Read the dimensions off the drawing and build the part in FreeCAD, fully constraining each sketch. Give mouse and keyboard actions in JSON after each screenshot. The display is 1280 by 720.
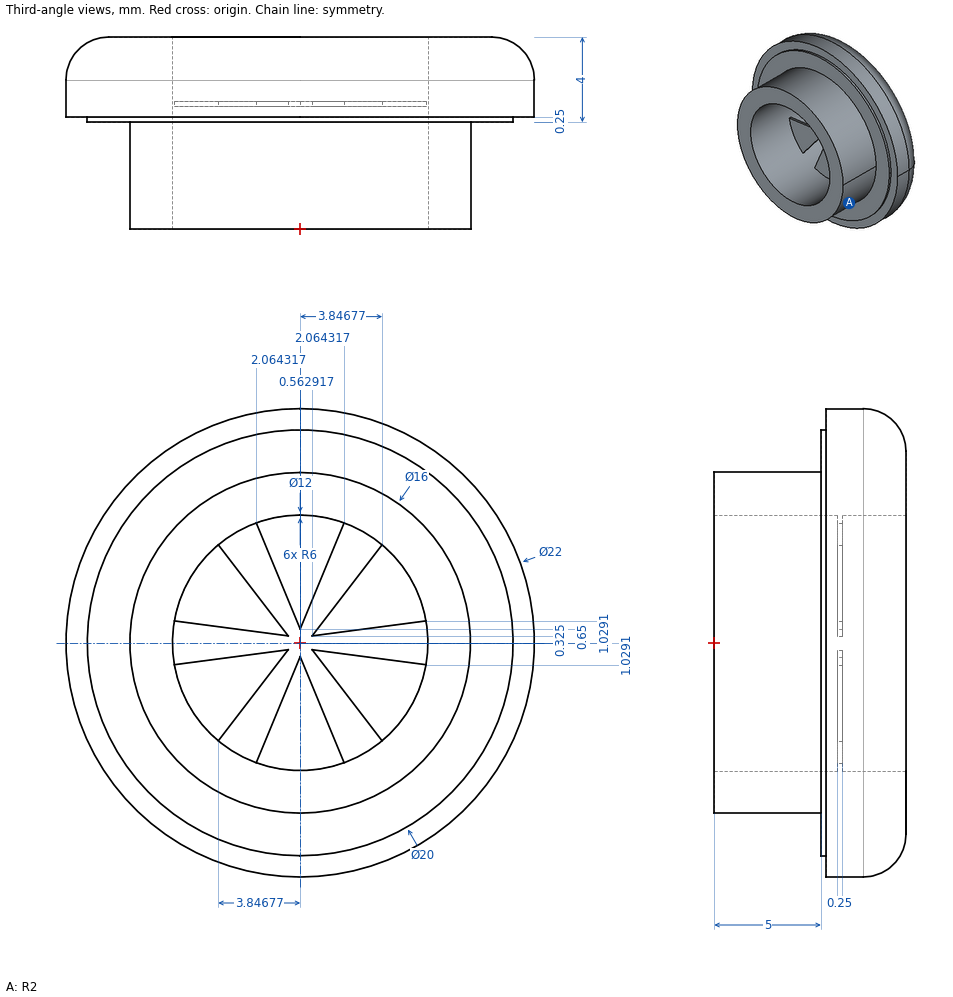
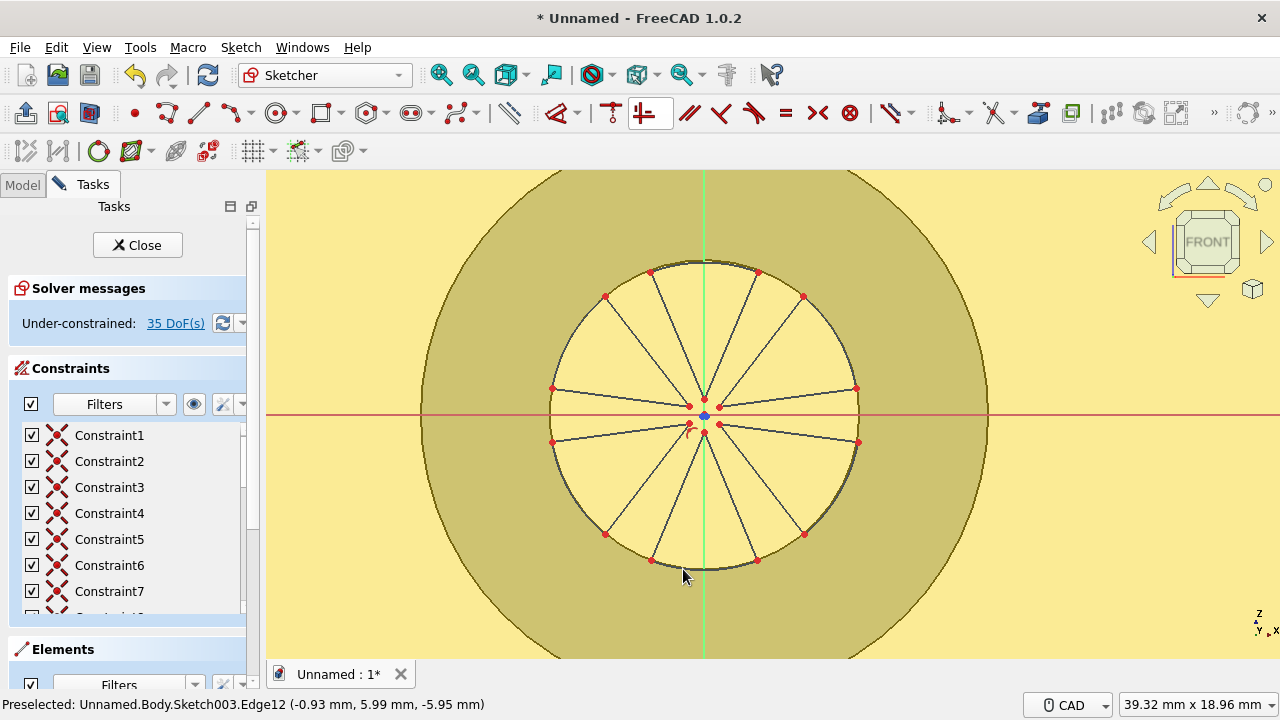
{"action": "left_click", "coordinate": [726, 264]}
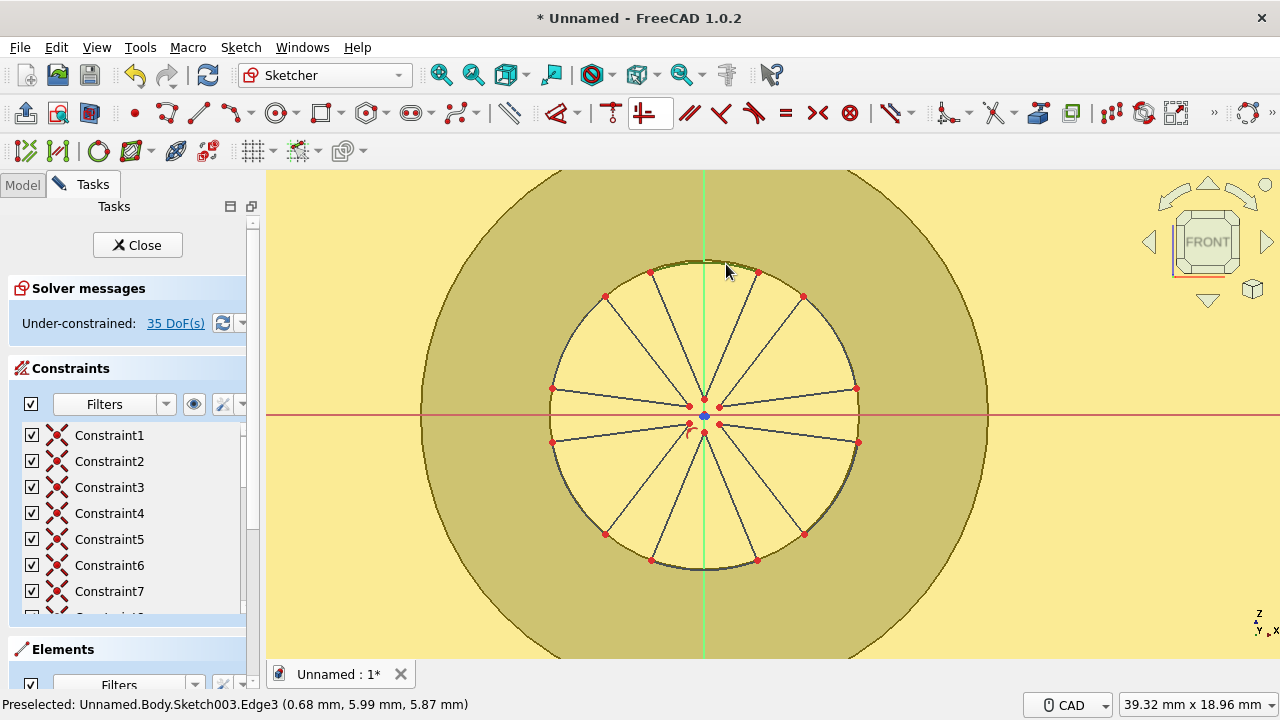
{"action": "left_click", "coordinate": [561, 473]}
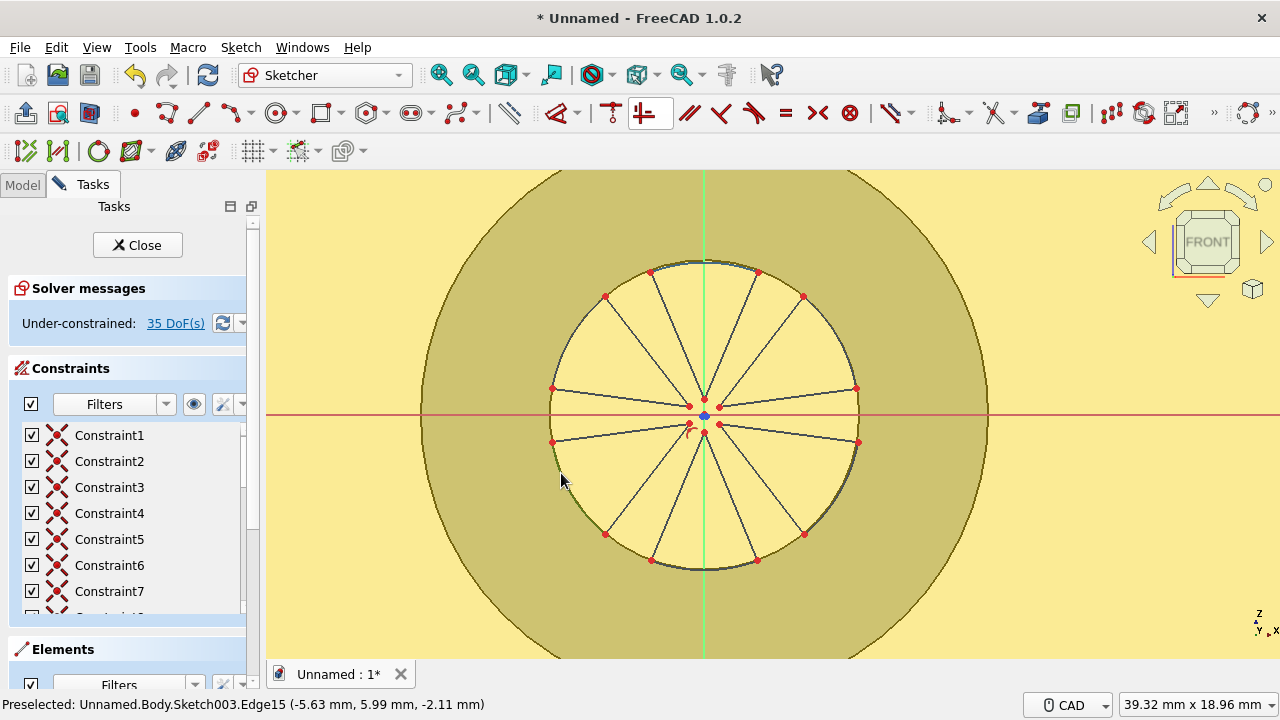
{"action": "left_click", "coordinate": [612, 114]}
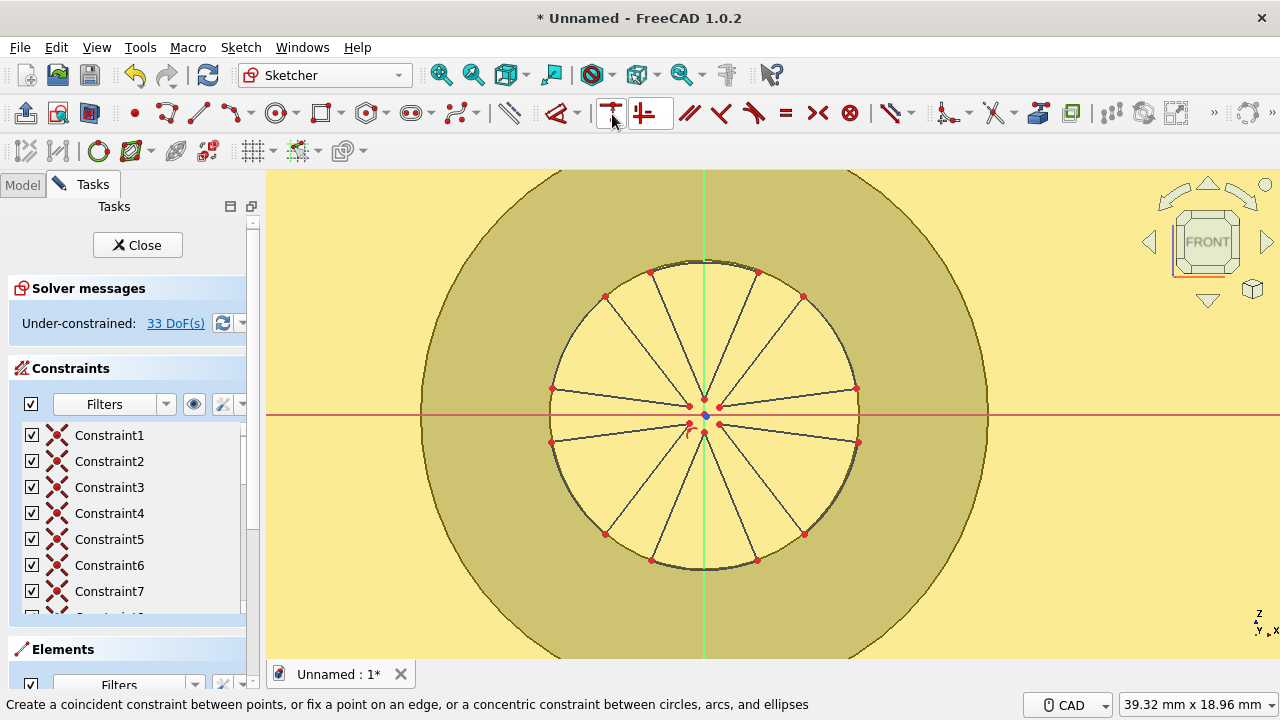
{"action": "left_click", "coordinate": [726, 264]}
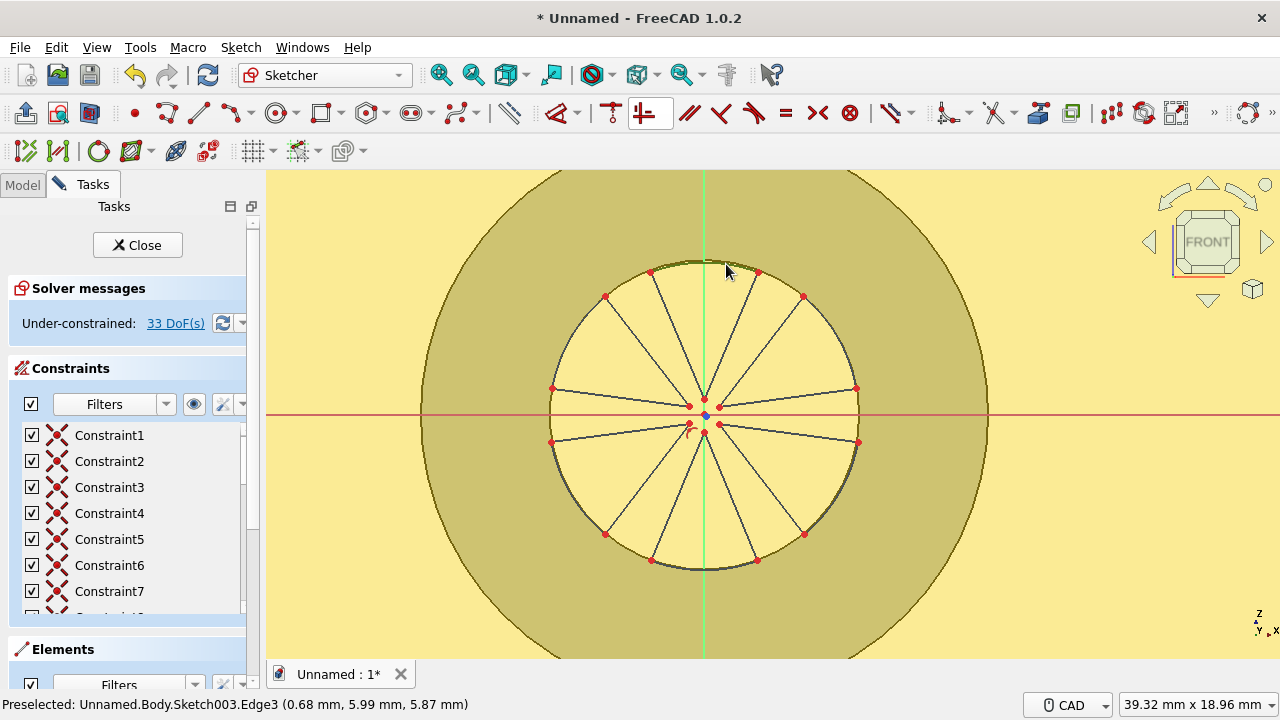
{"action": "left_click", "coordinate": [583, 320]}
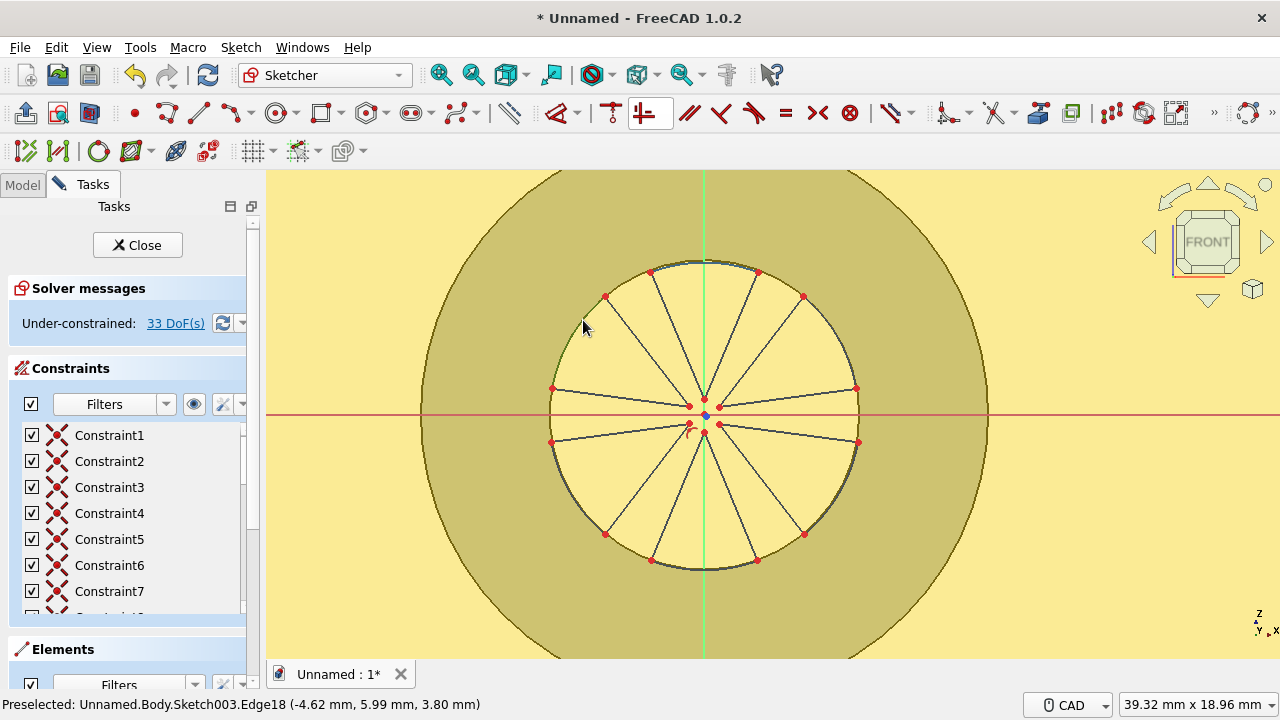
{"action": "left_click", "coordinate": [612, 114]}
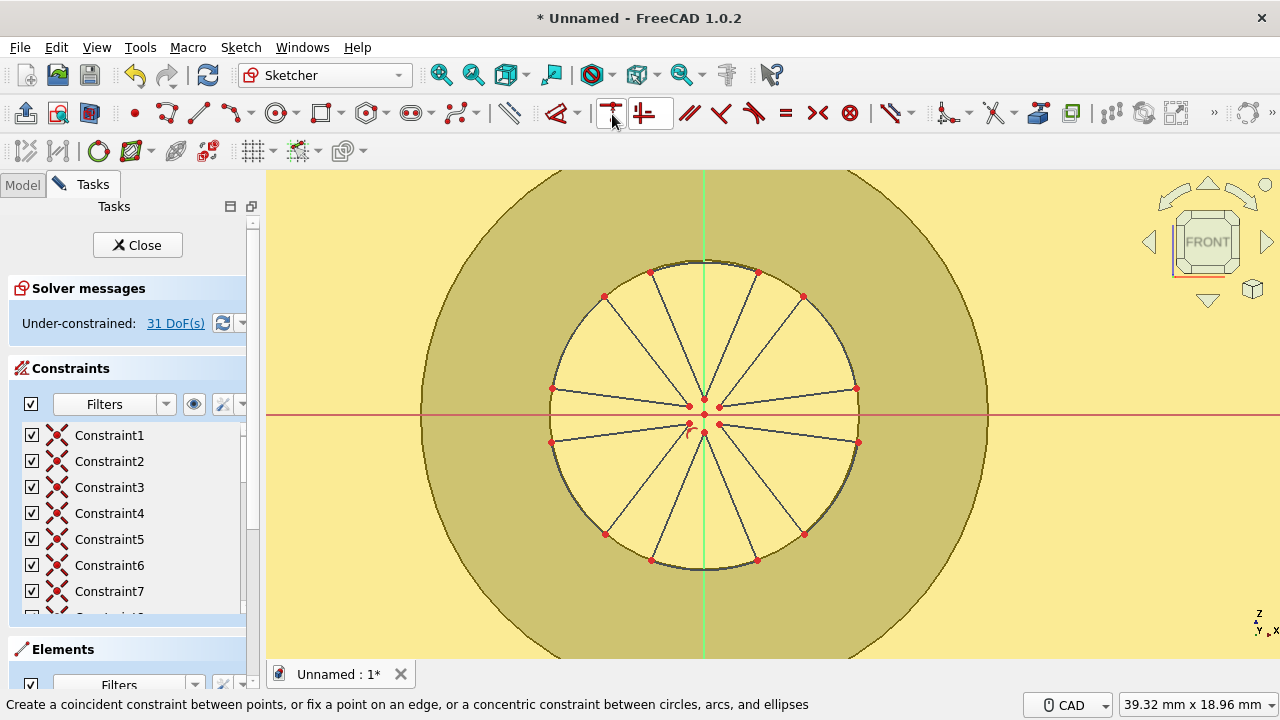
{"action": "scroll", "coordinate": [704, 415], "scroll_direction": "up", "scroll_amount": 5}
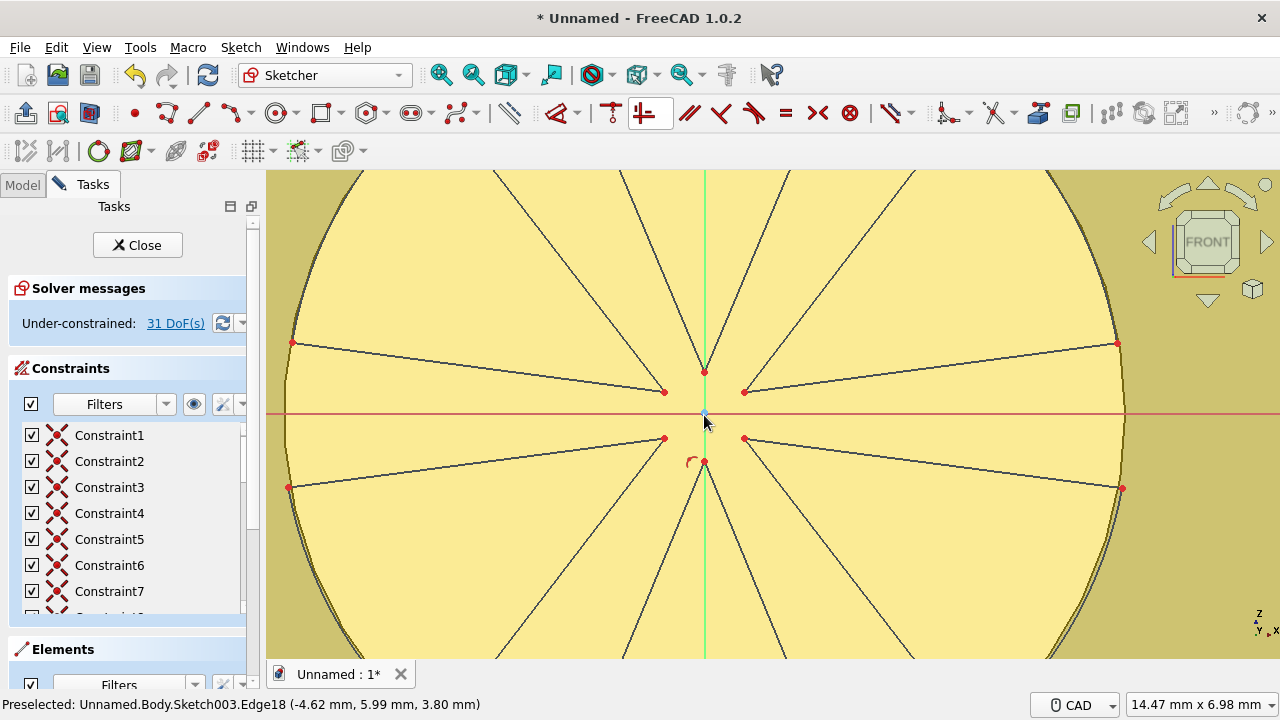
{"action": "left_click_drag", "start_coordinate": [694, 402], "coordinate": [715, 424]}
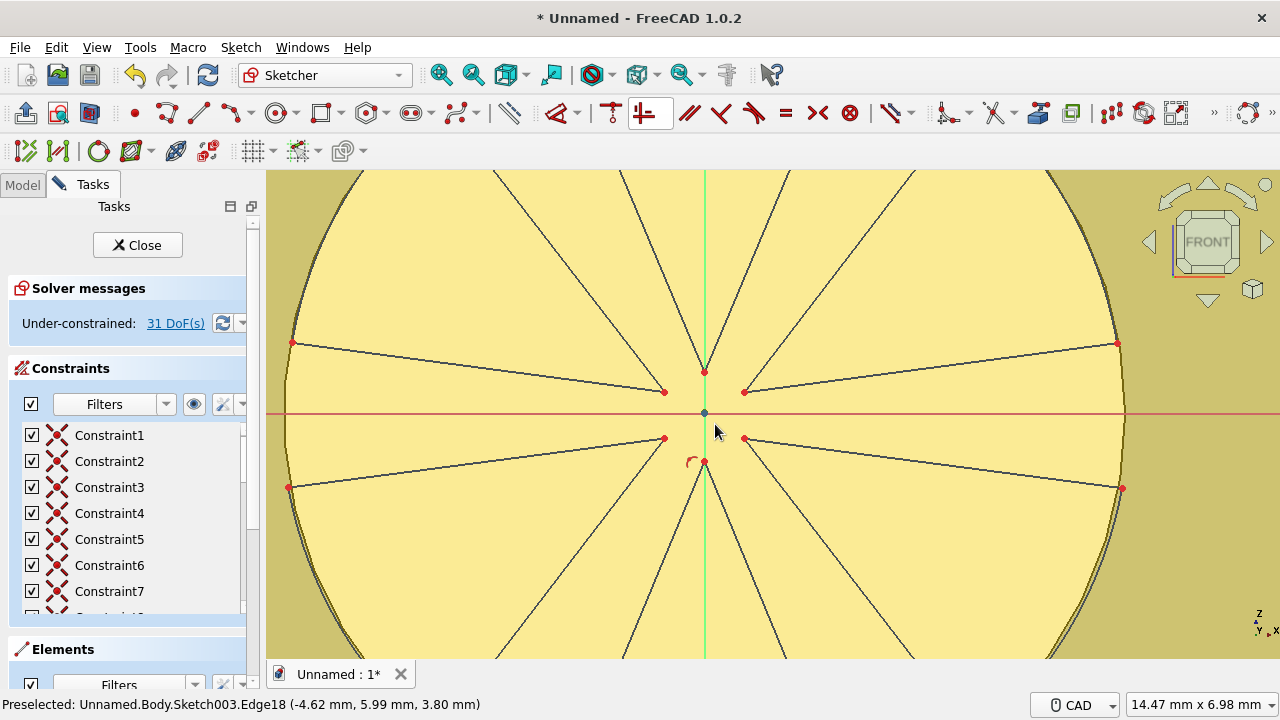
{"action": "left_click", "coordinate": [612, 114]}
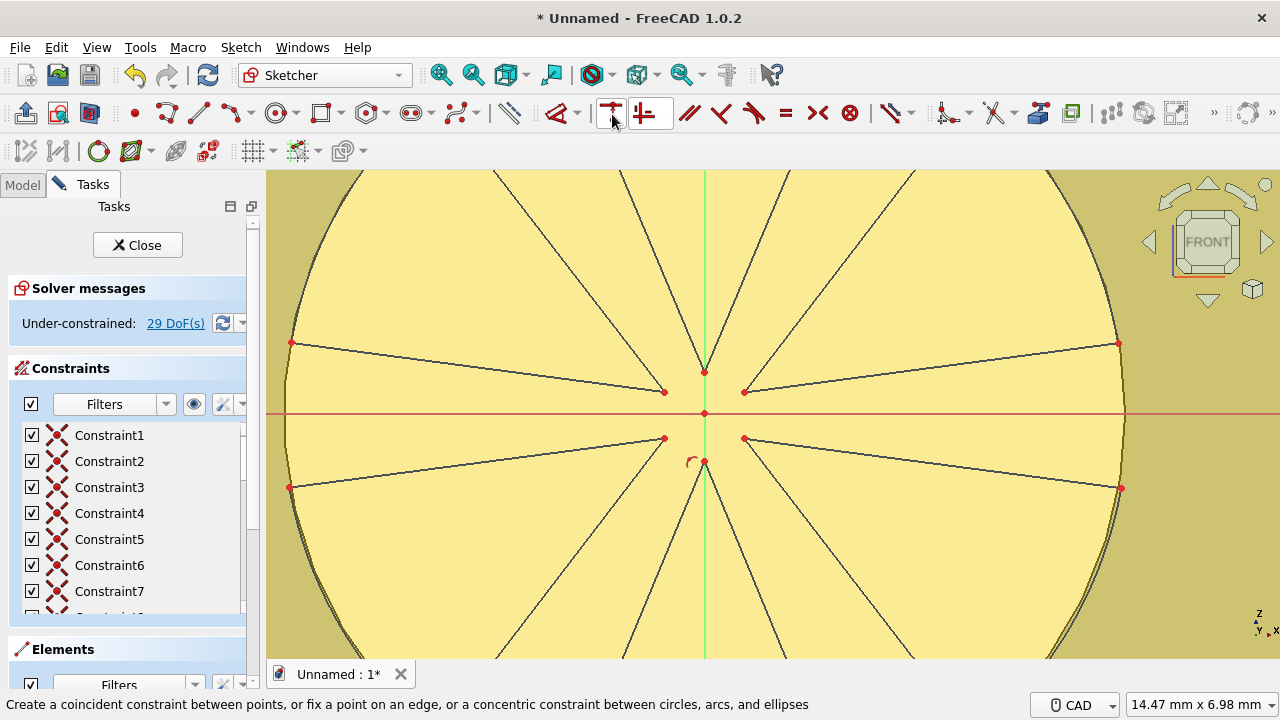
{"action": "scroll", "coordinate": [704, 415], "scroll_direction": "down", "scroll_amount": 5}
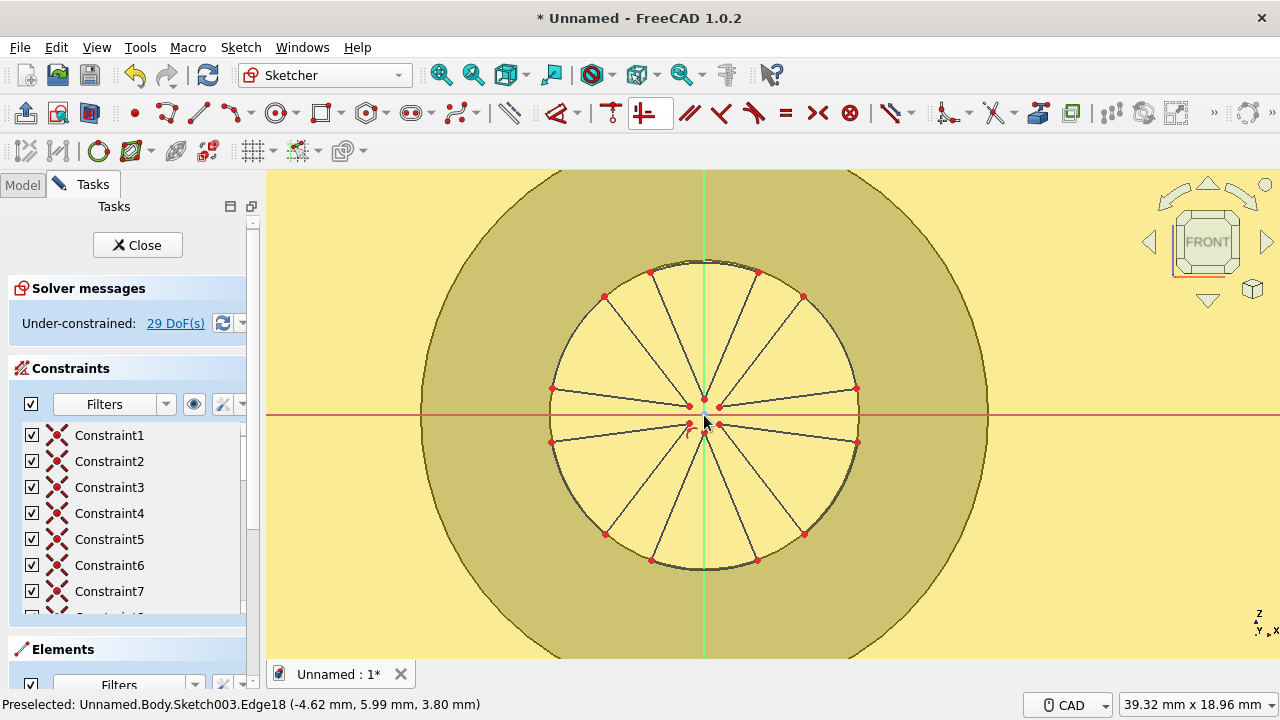
{"action": "left_click", "coordinate": [726, 264]}